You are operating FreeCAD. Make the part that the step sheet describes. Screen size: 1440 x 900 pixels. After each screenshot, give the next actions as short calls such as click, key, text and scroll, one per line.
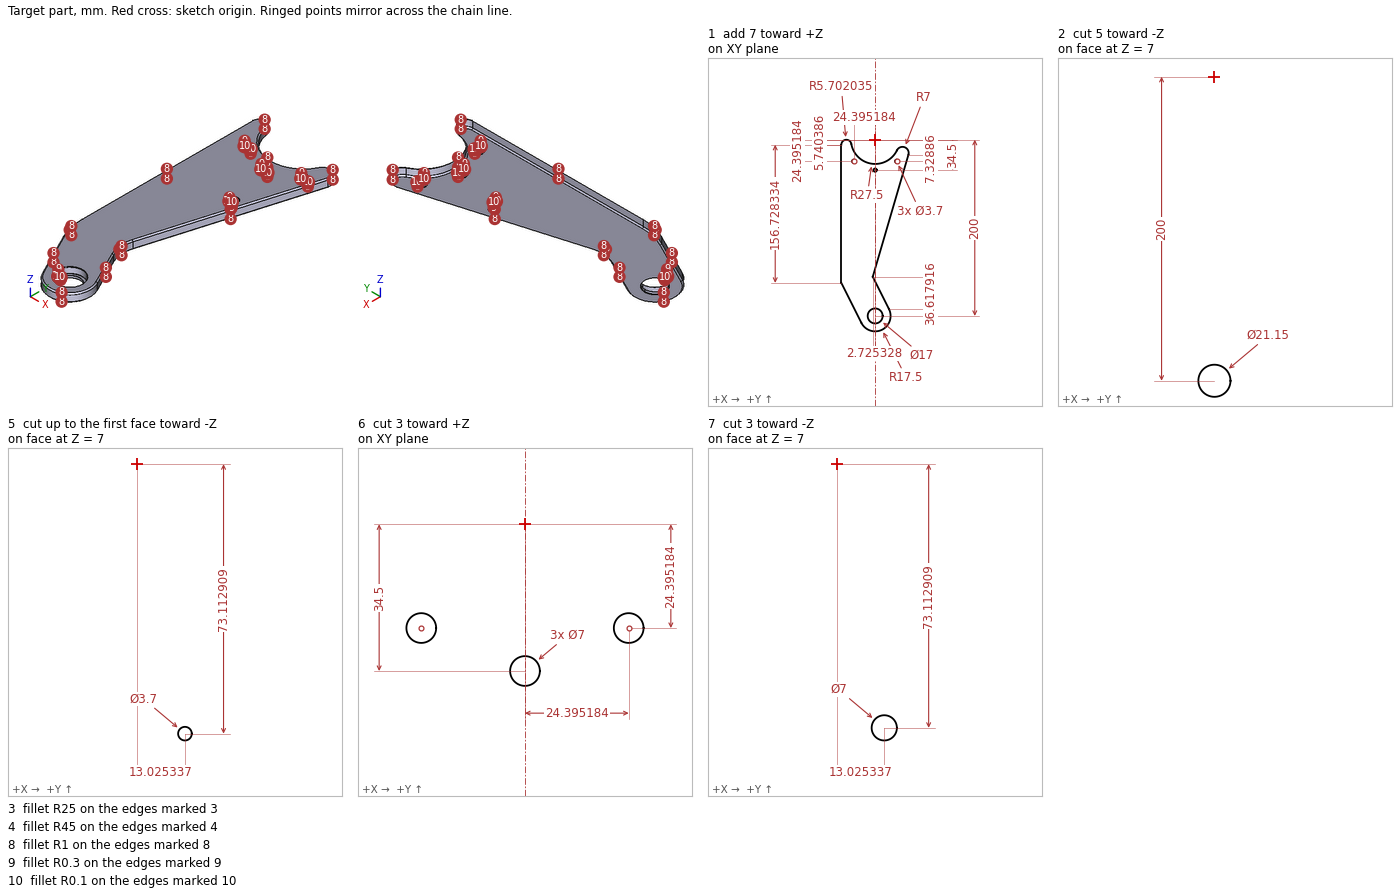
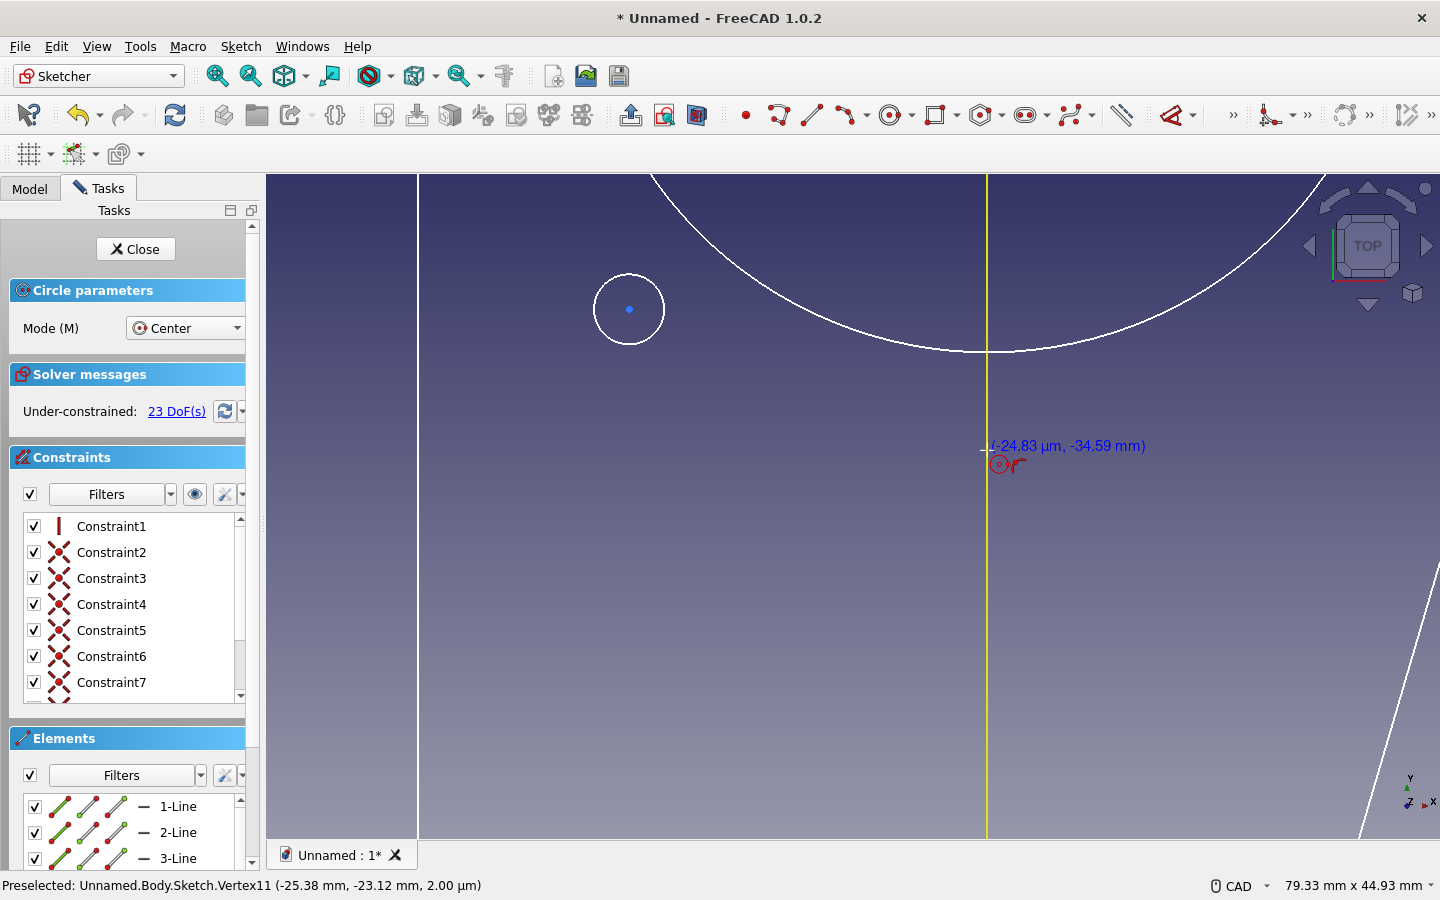
scroll(754, 346, down, 10)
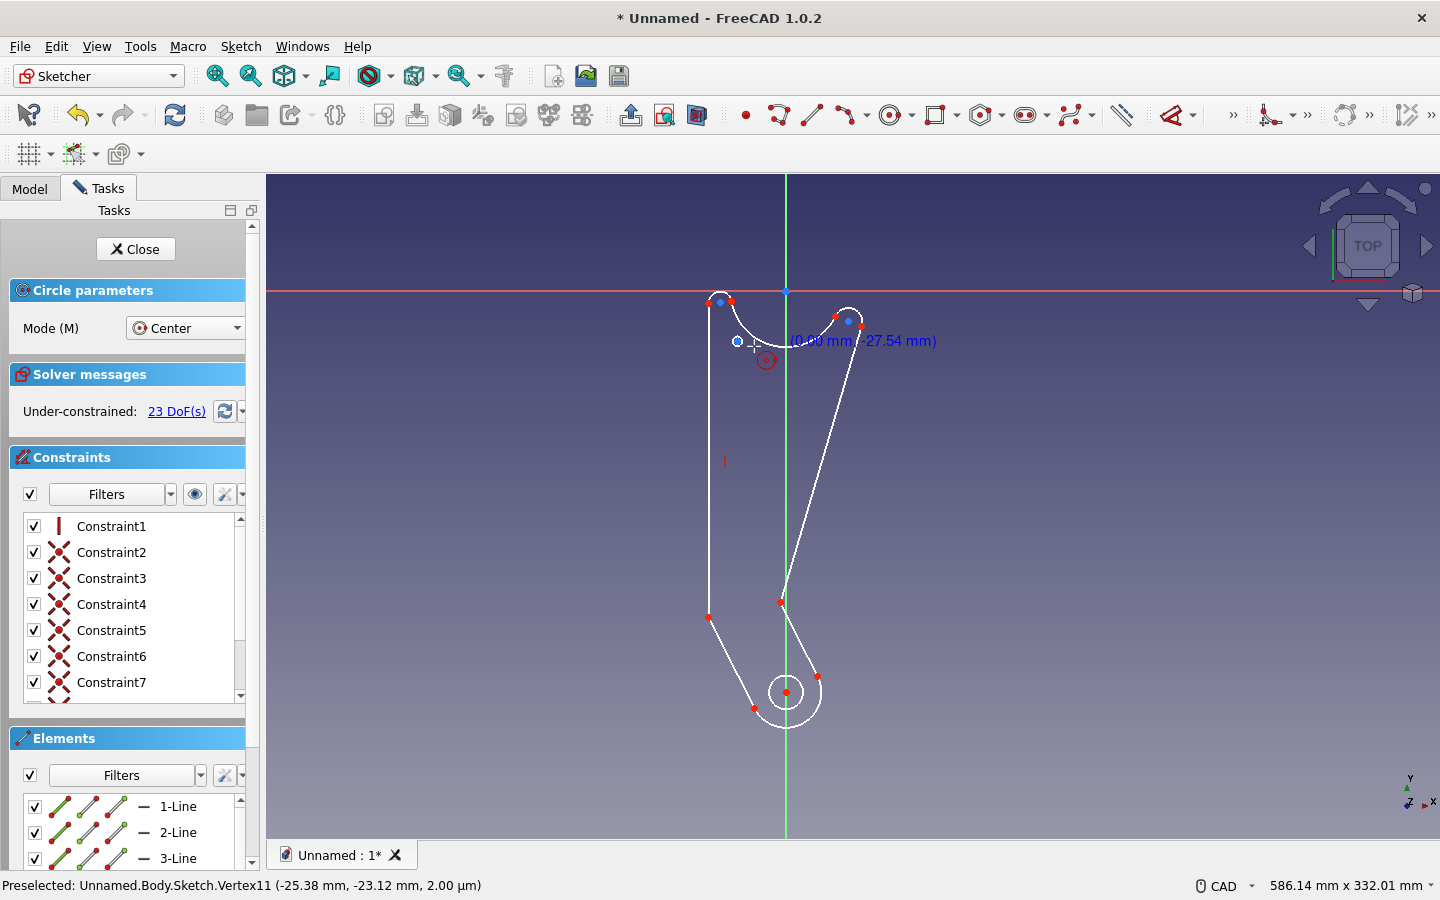
click(786, 360)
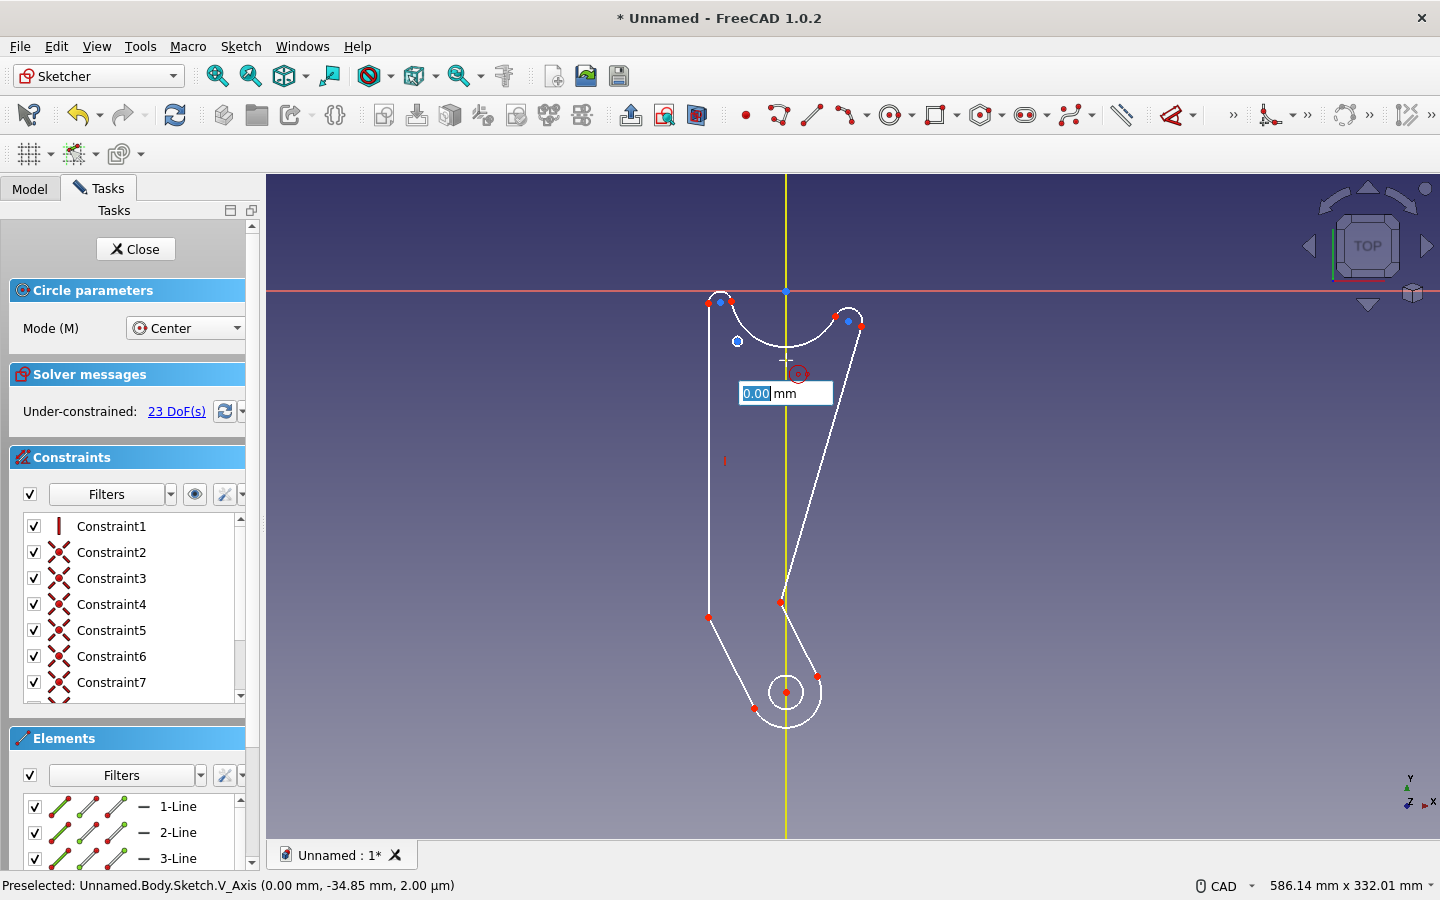
scroll(789, 359, up, 8)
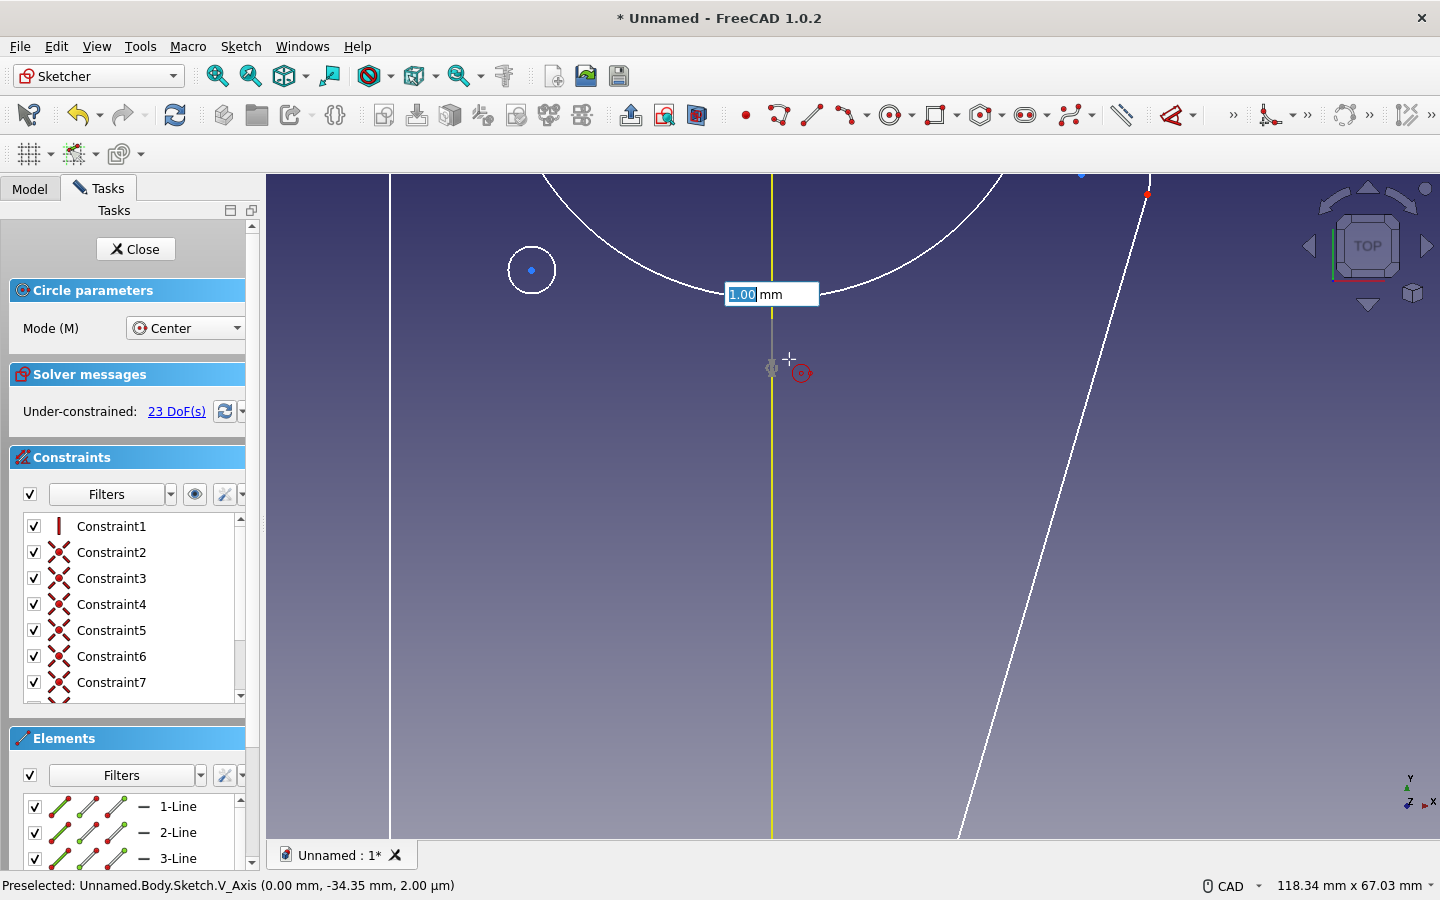
click(789, 358)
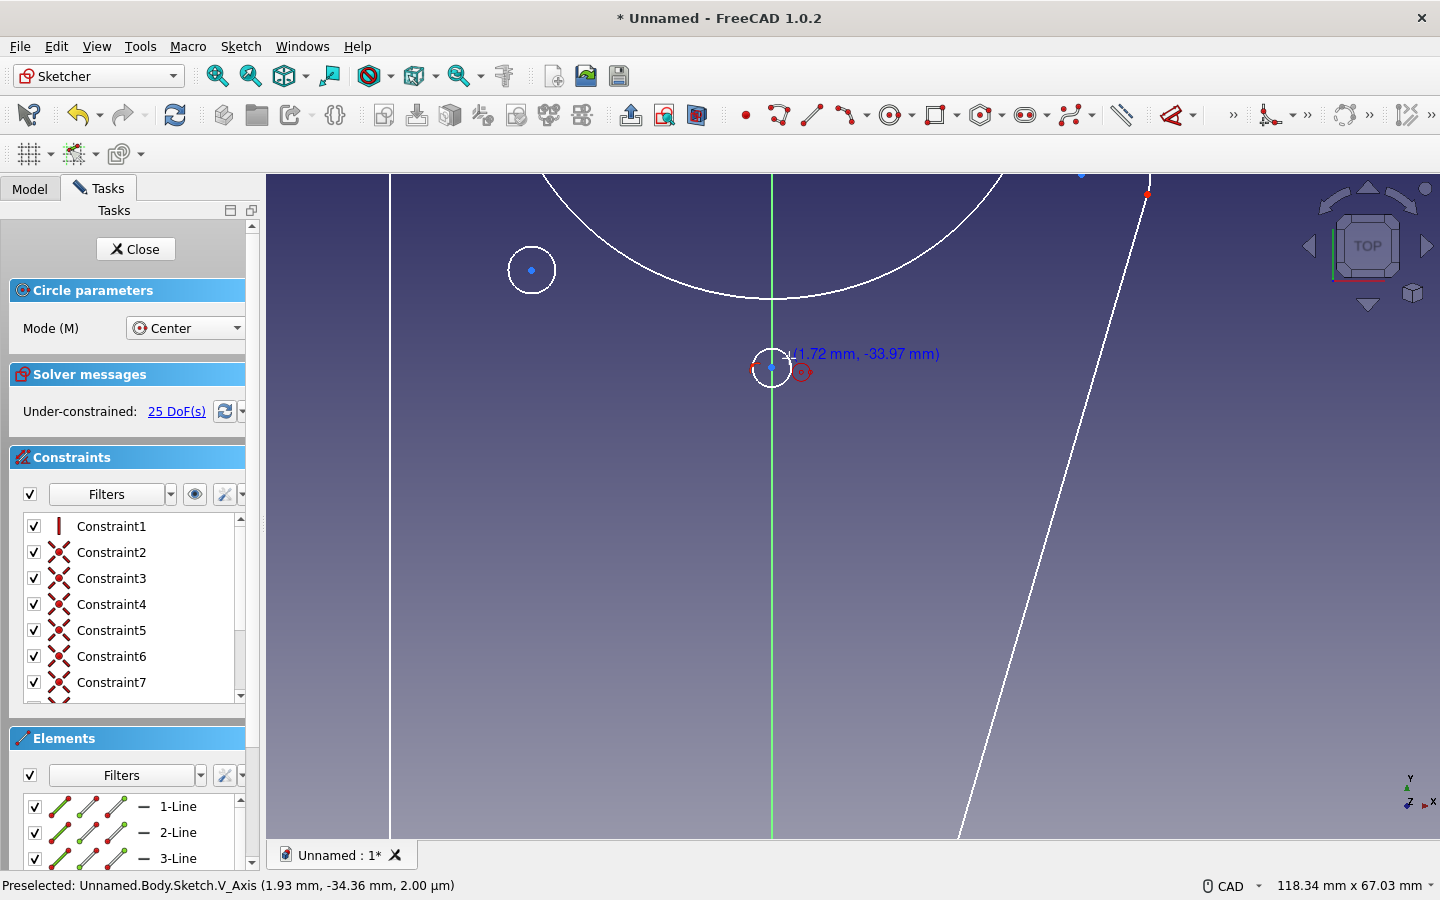
scroll(1014, 264, up, 2)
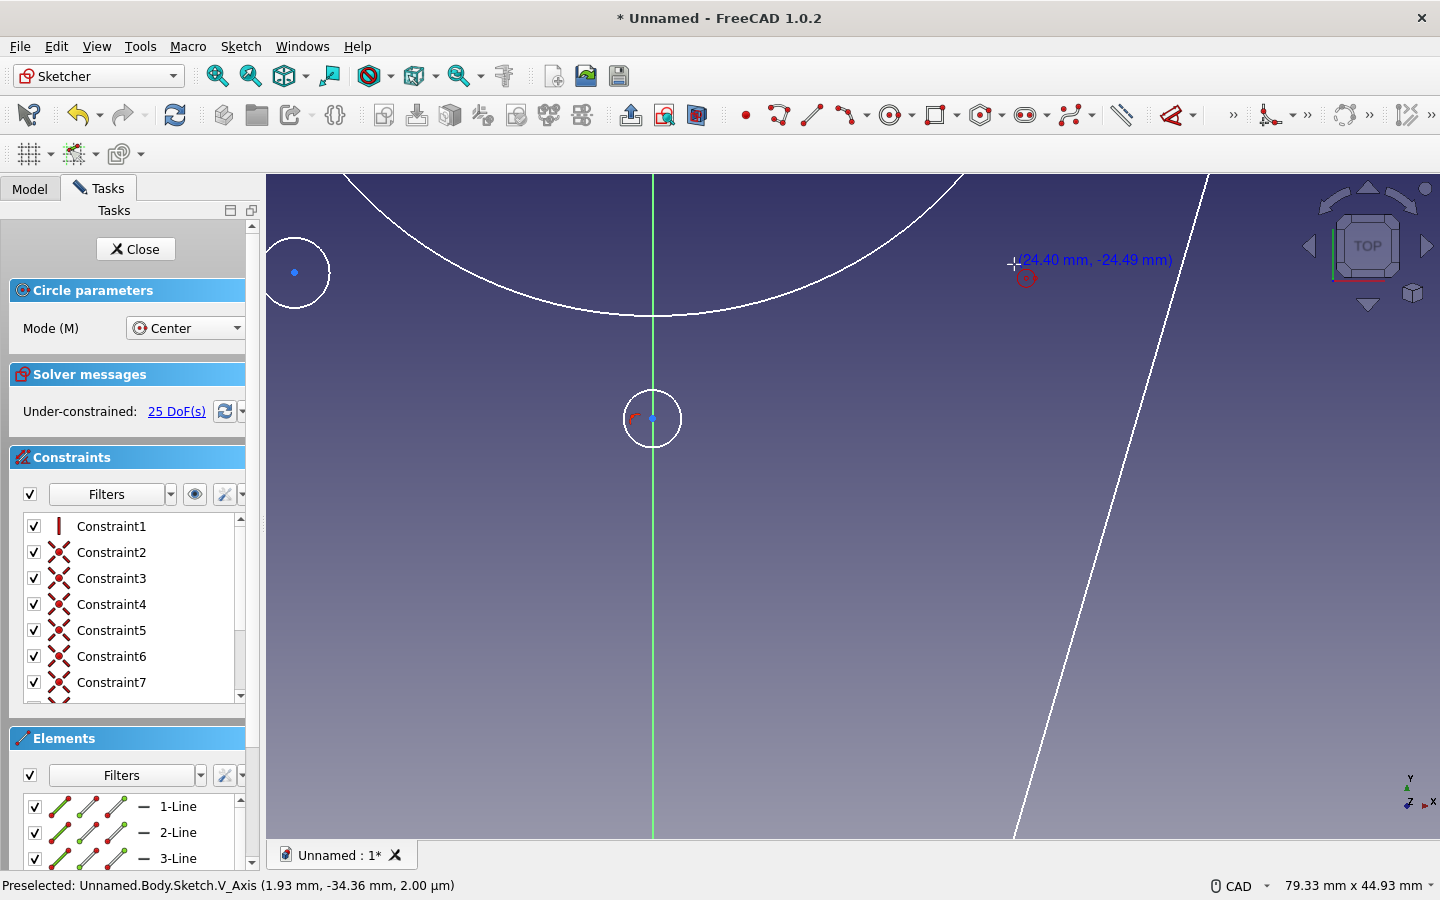
scroll(806, 351, down, 10)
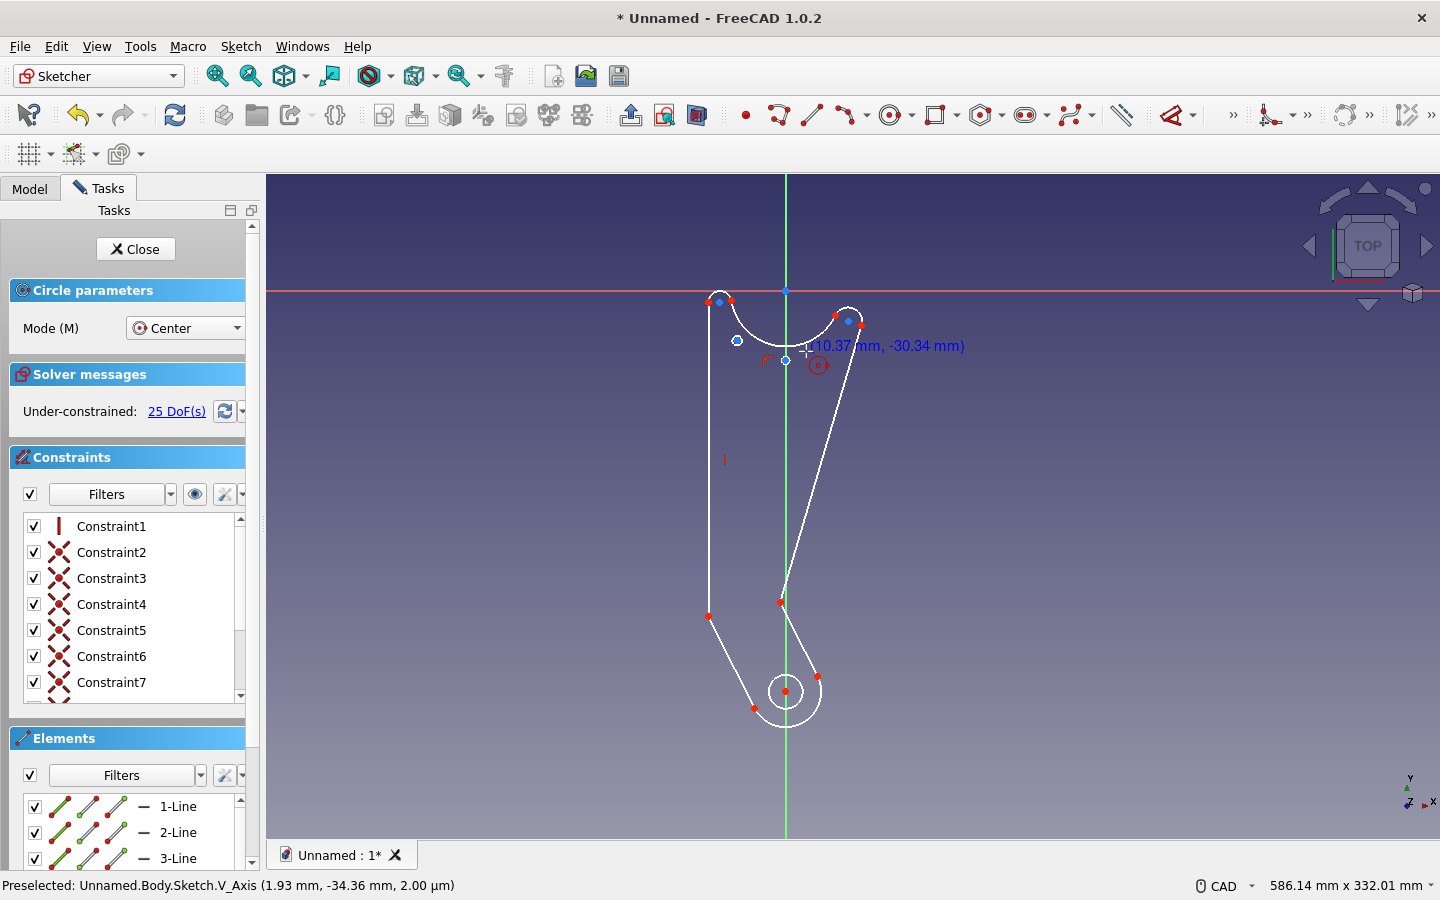
click(834, 339)